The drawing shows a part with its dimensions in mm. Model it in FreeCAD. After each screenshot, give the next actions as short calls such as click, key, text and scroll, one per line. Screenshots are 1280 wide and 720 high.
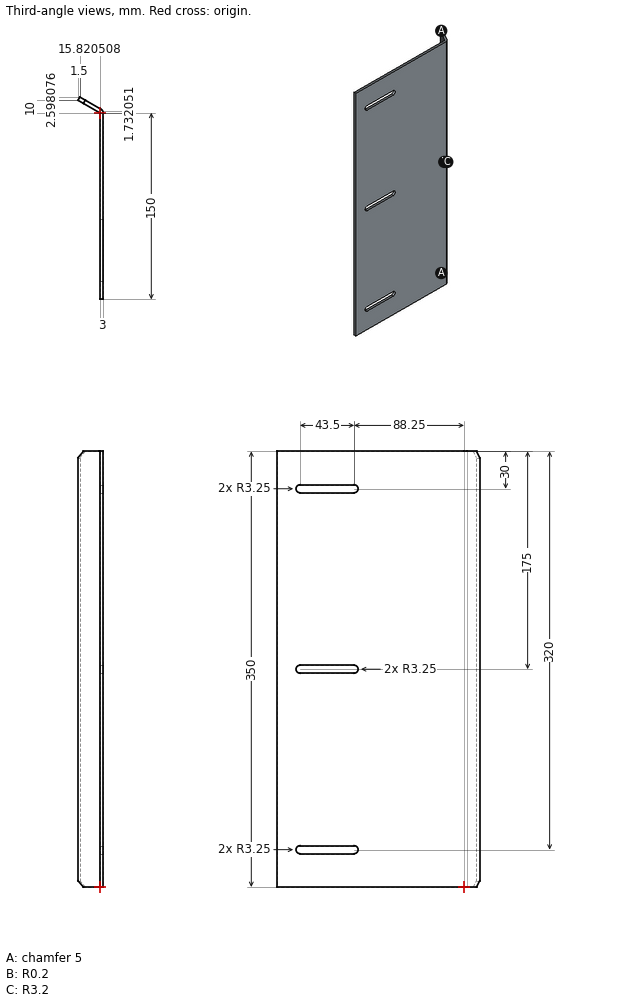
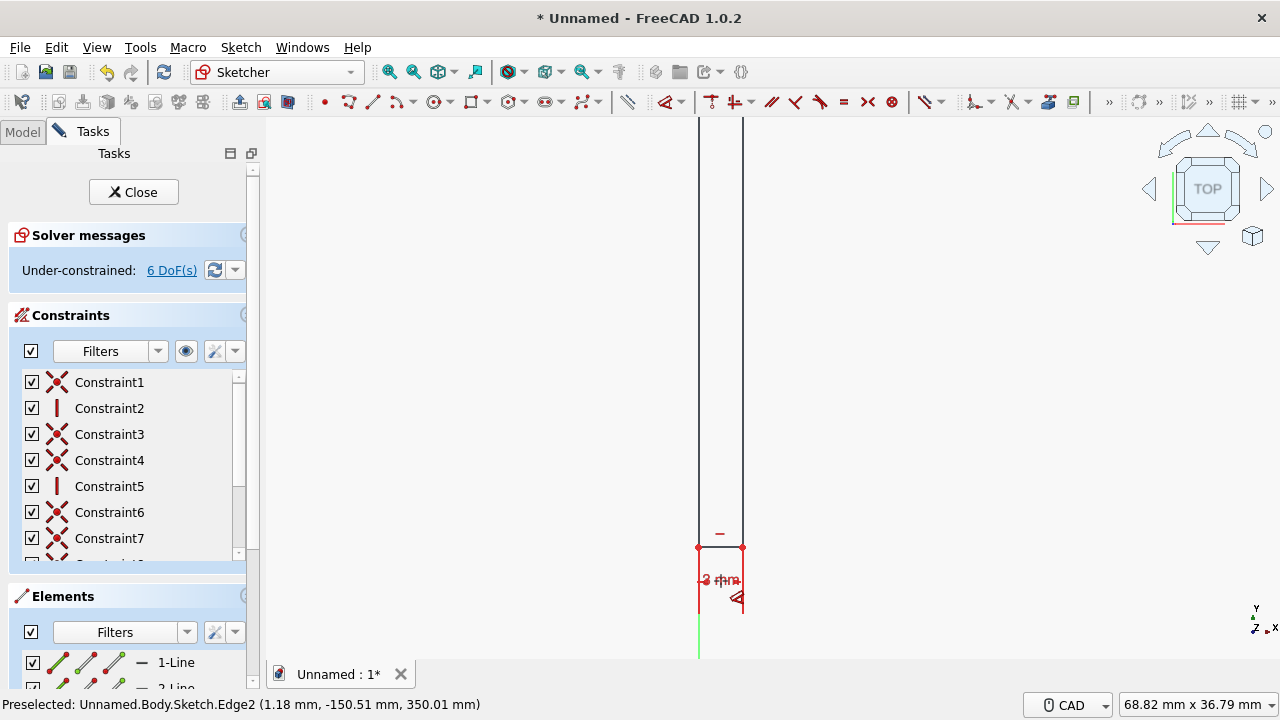
scroll(722, 552, down, 10)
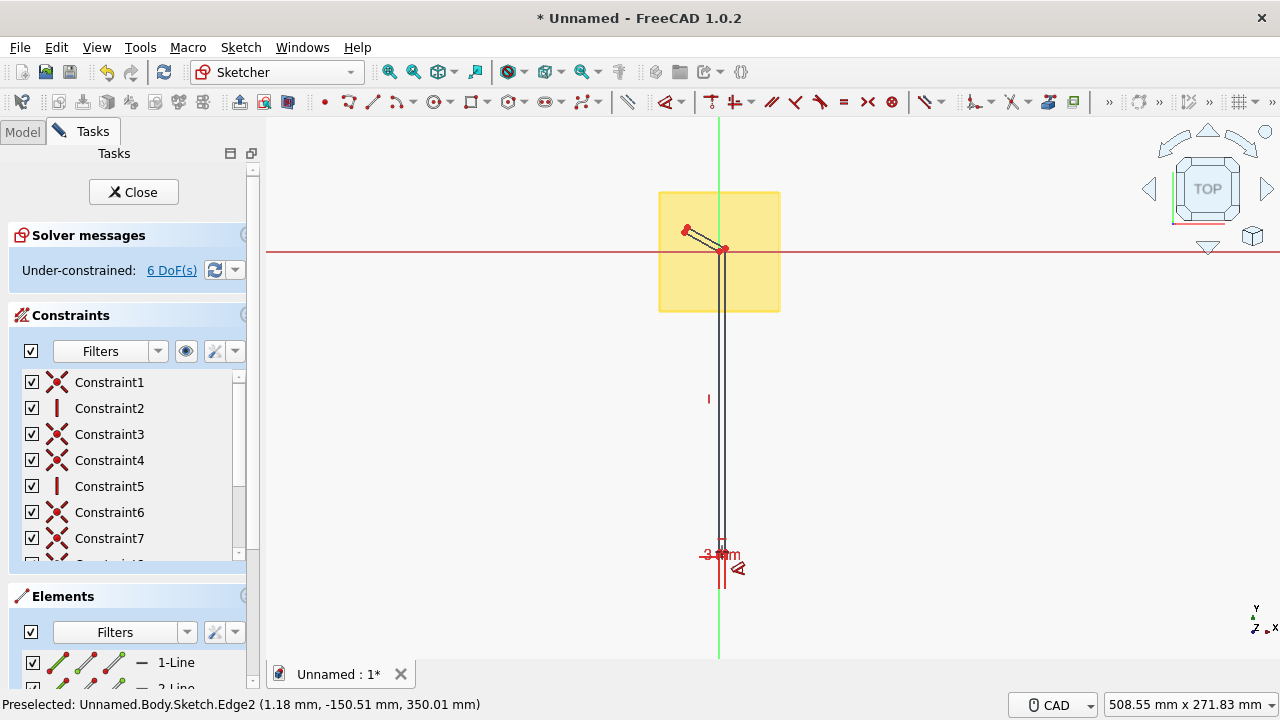
scroll(719, 342, up, 5)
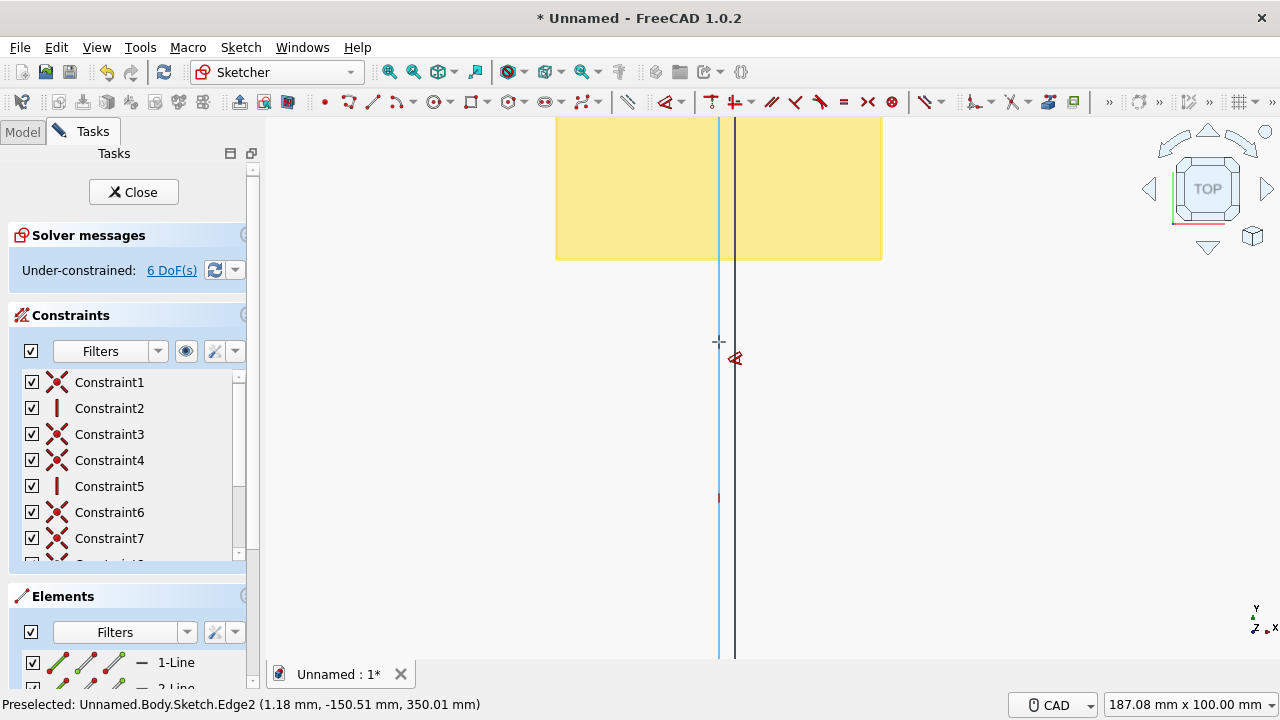
click(719, 341)
click(753, 388)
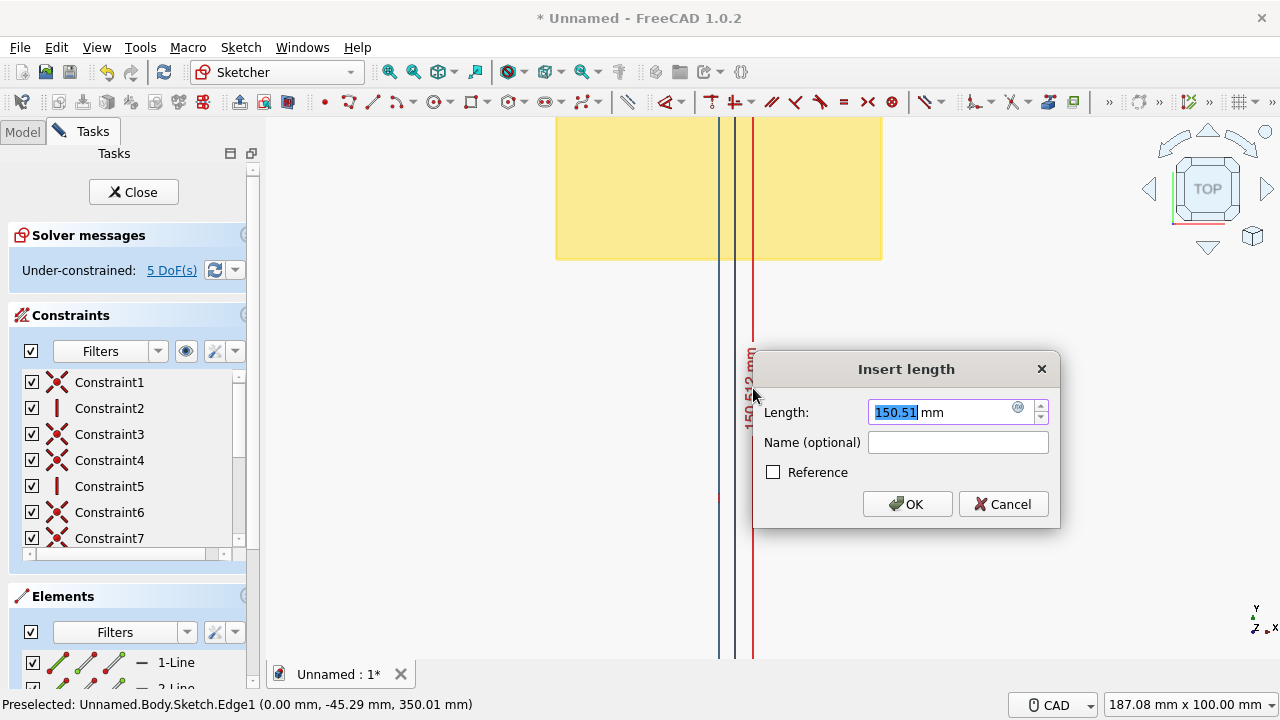
text(150)
key(Return)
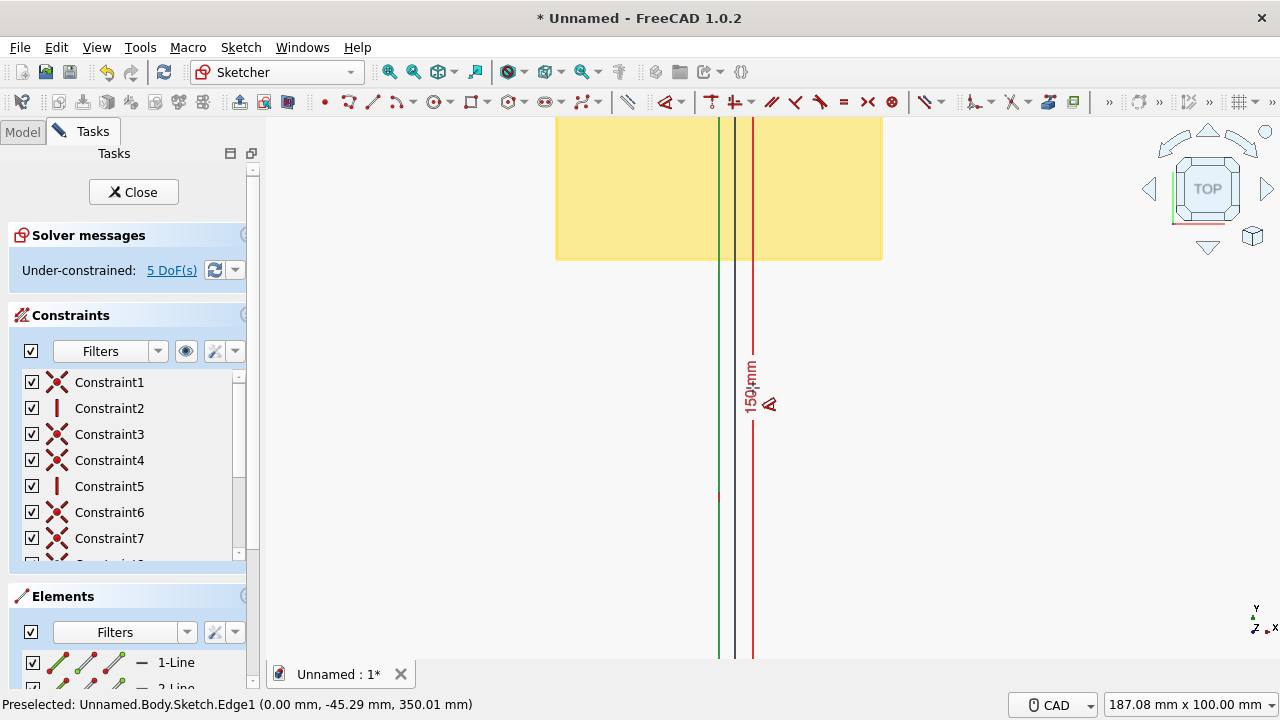
scroll(719, 341, down, 5)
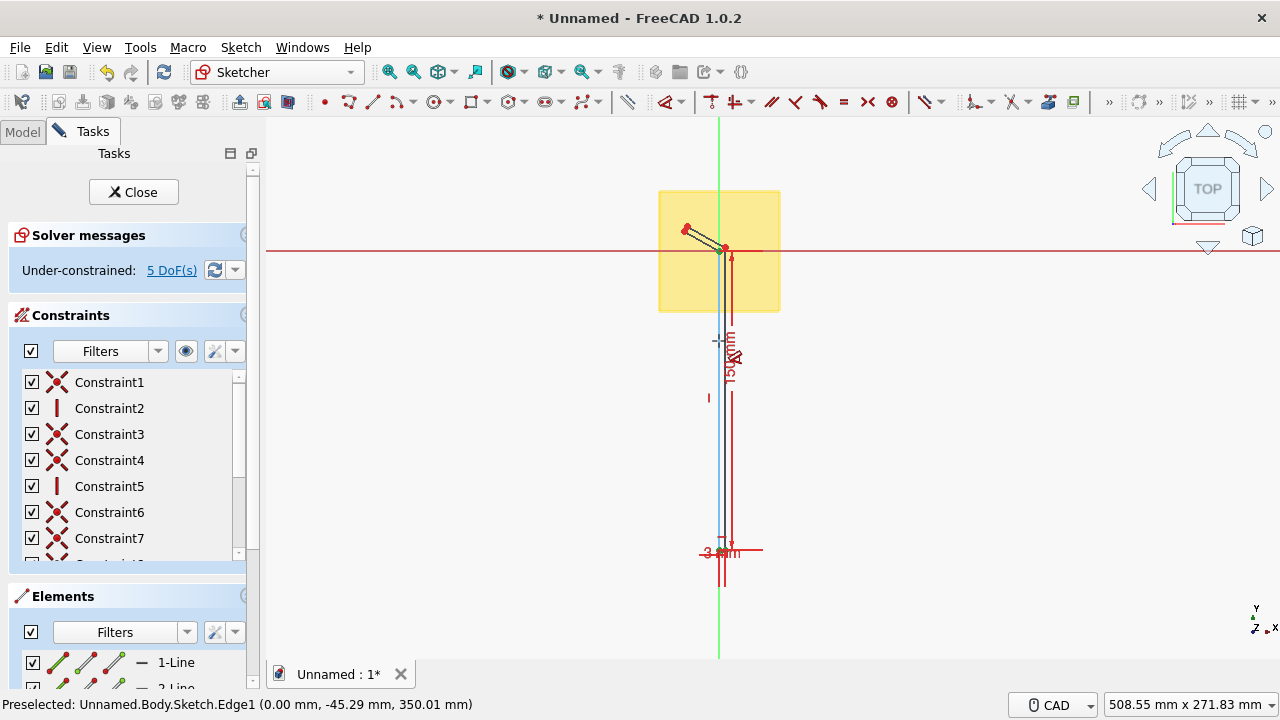
scroll(685, 232, up, 4)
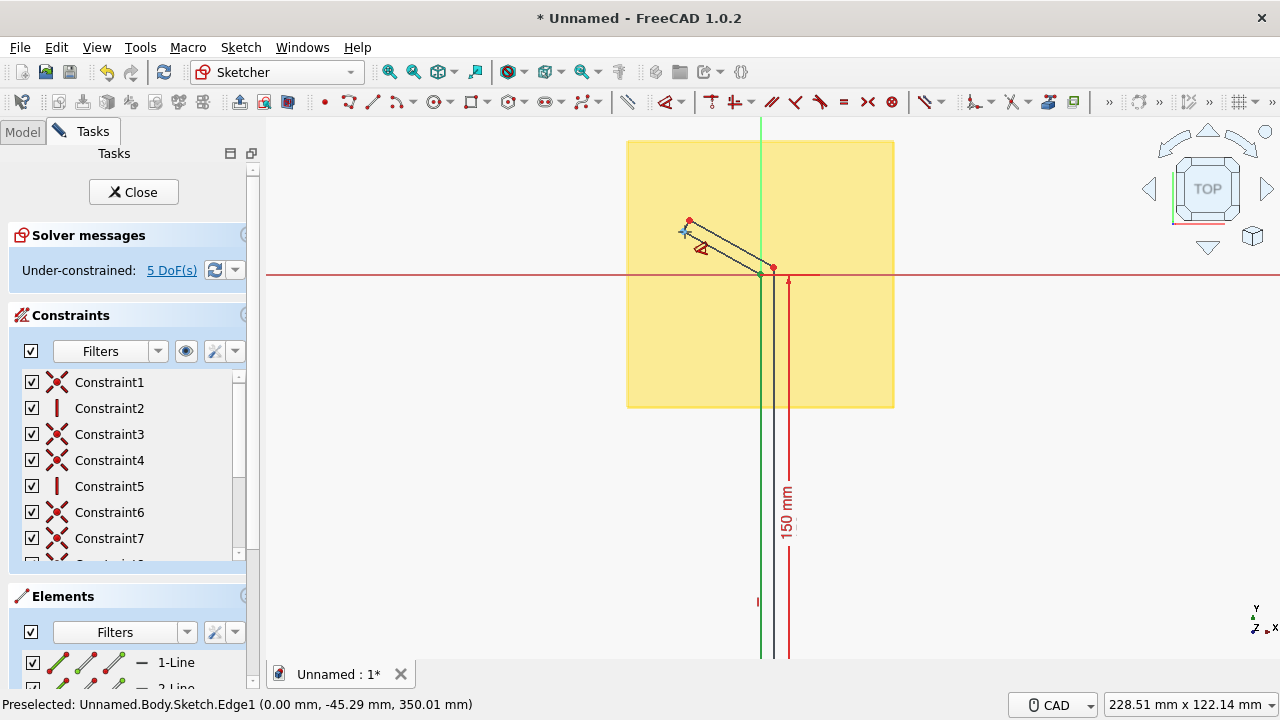
click(684, 232)
click(650, 253)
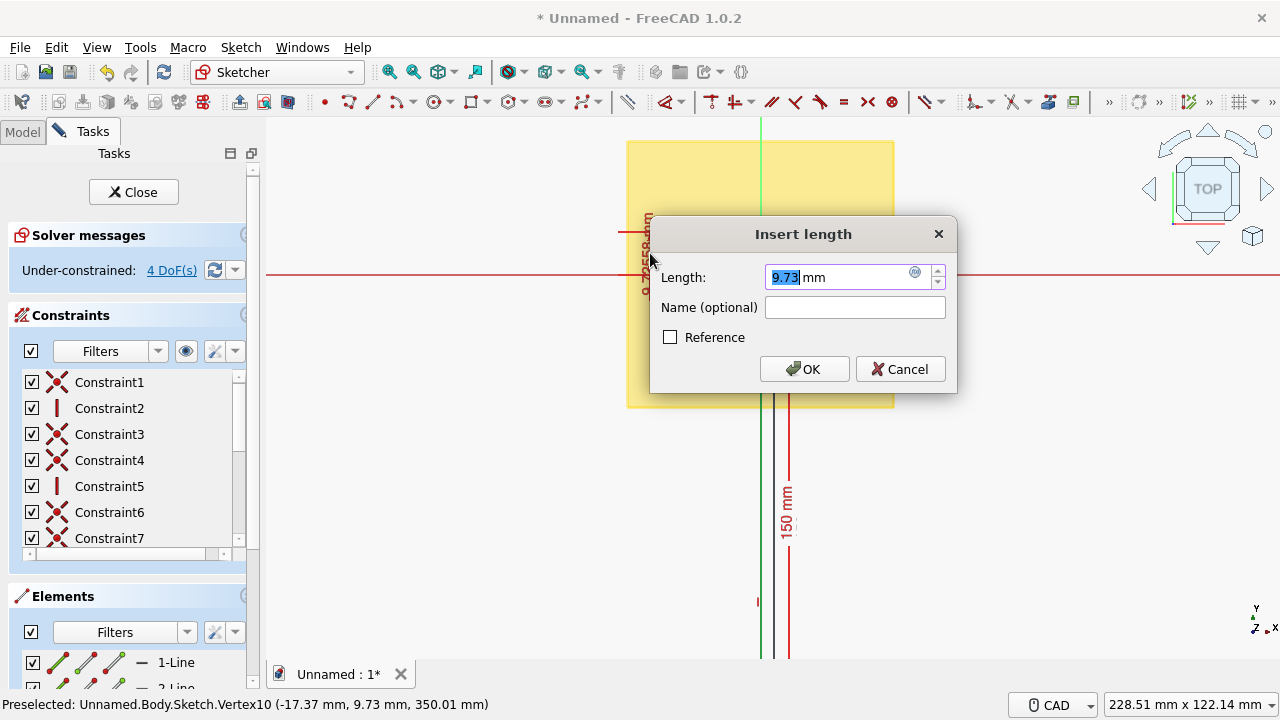
text(10)
key(Return)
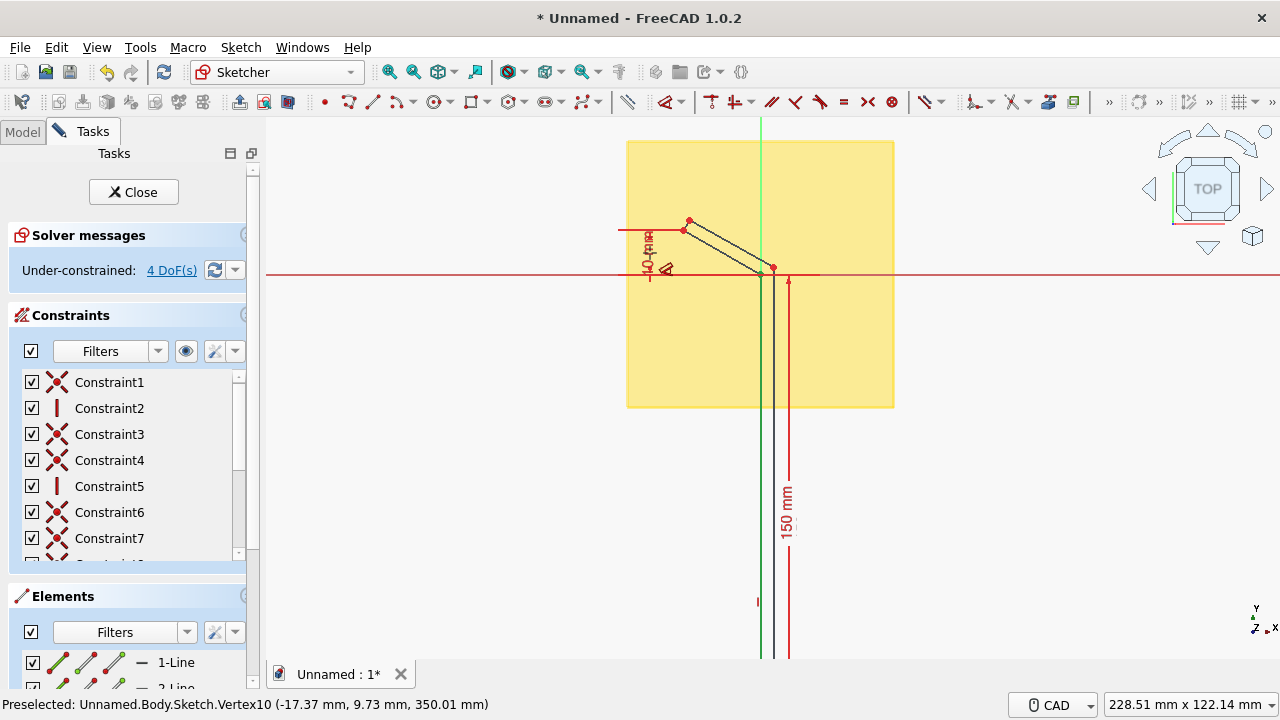
scroll(687, 225, up, 9)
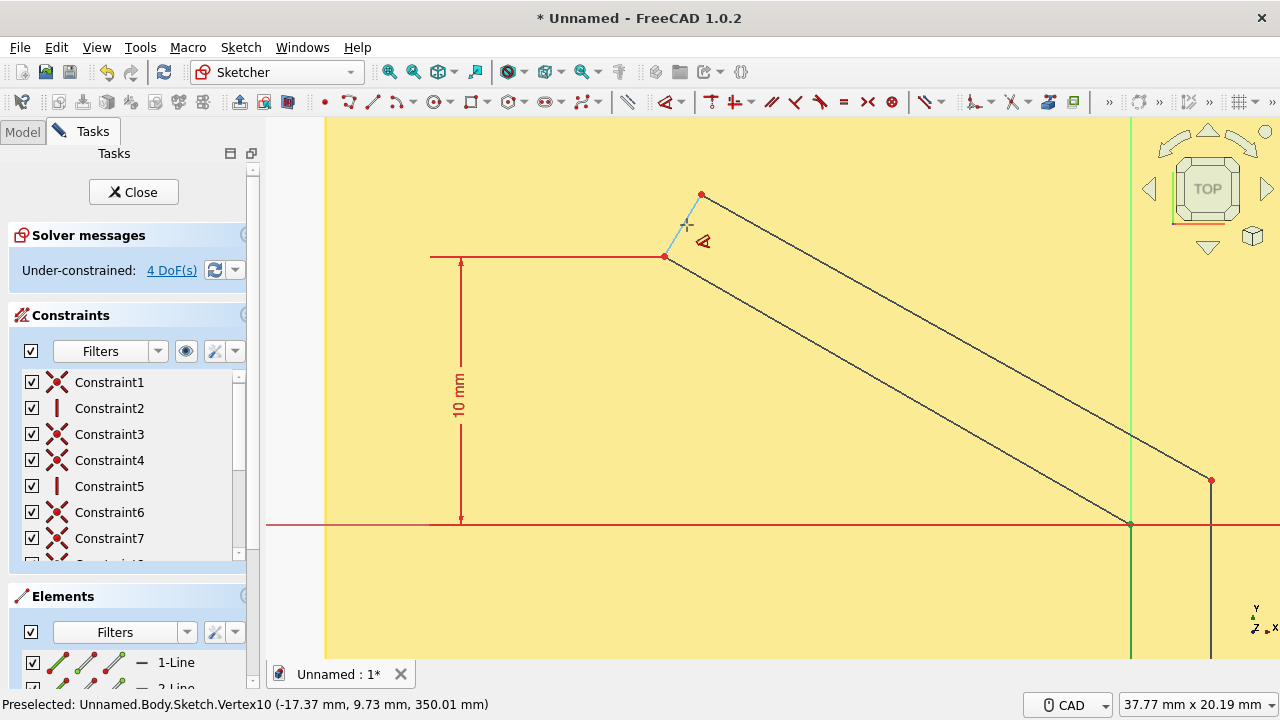
click(683, 226)
click(683, 161)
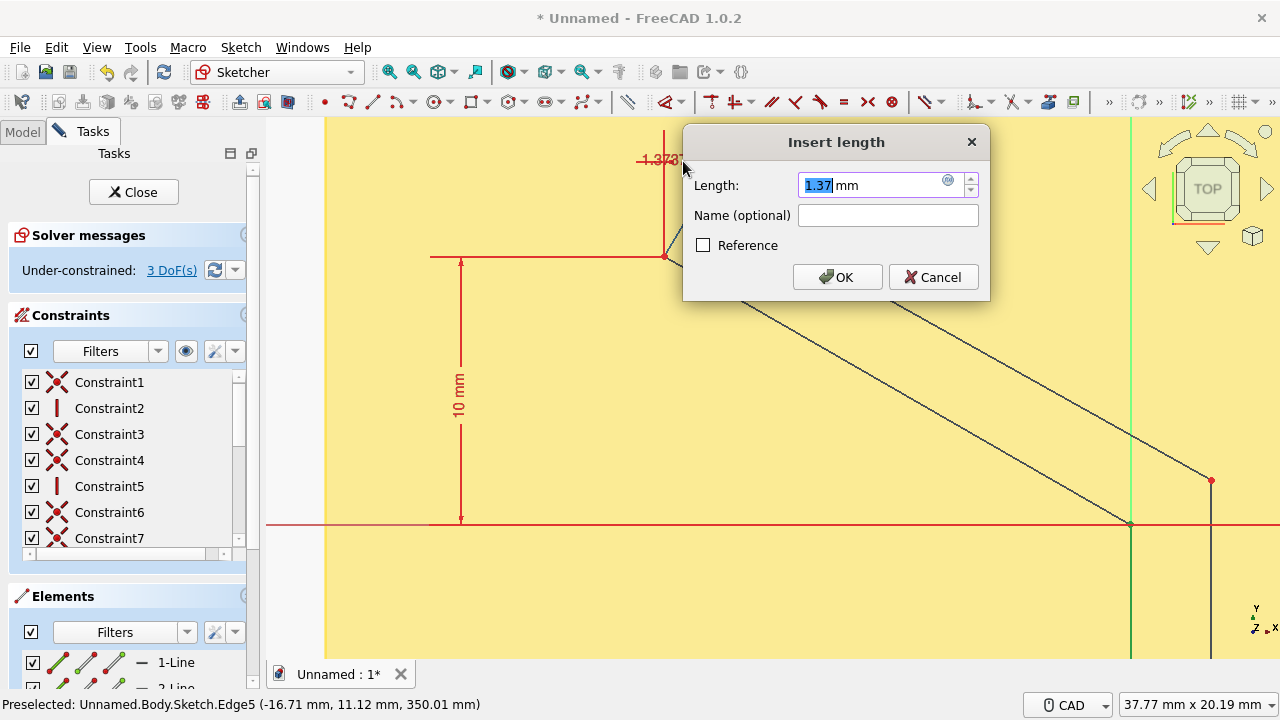
text(1.5)
key(Return)